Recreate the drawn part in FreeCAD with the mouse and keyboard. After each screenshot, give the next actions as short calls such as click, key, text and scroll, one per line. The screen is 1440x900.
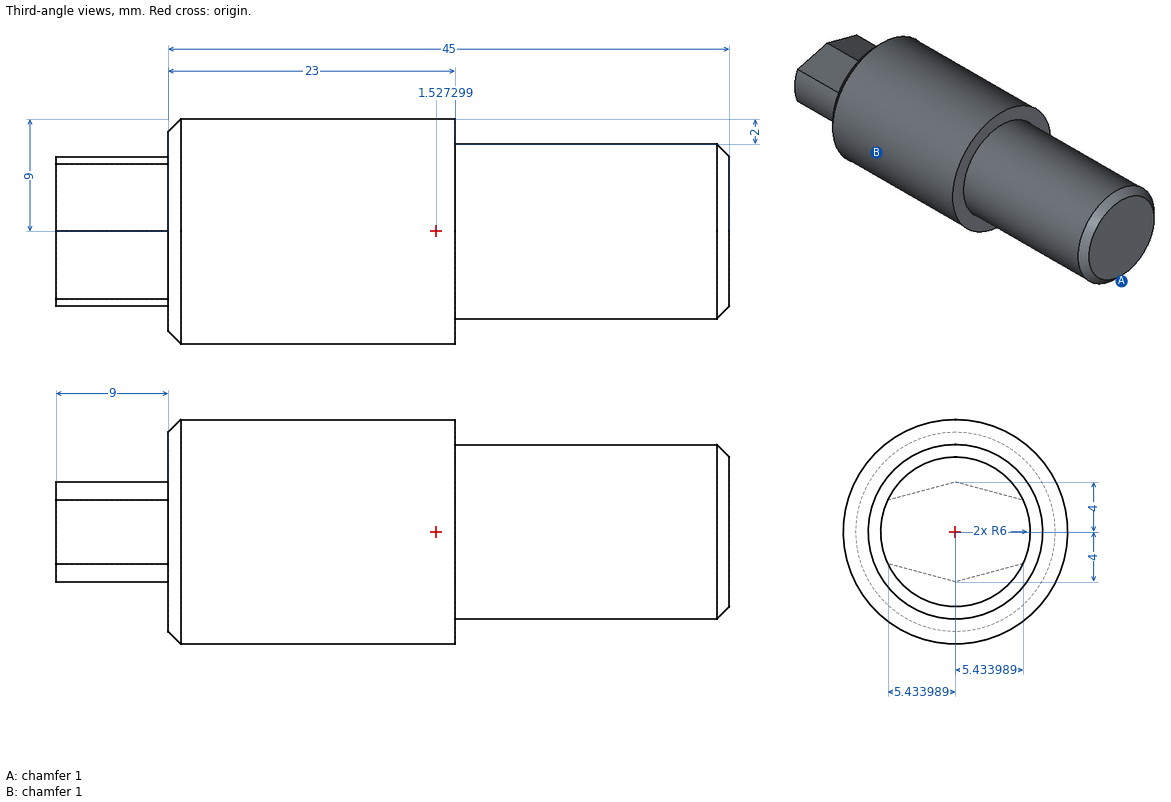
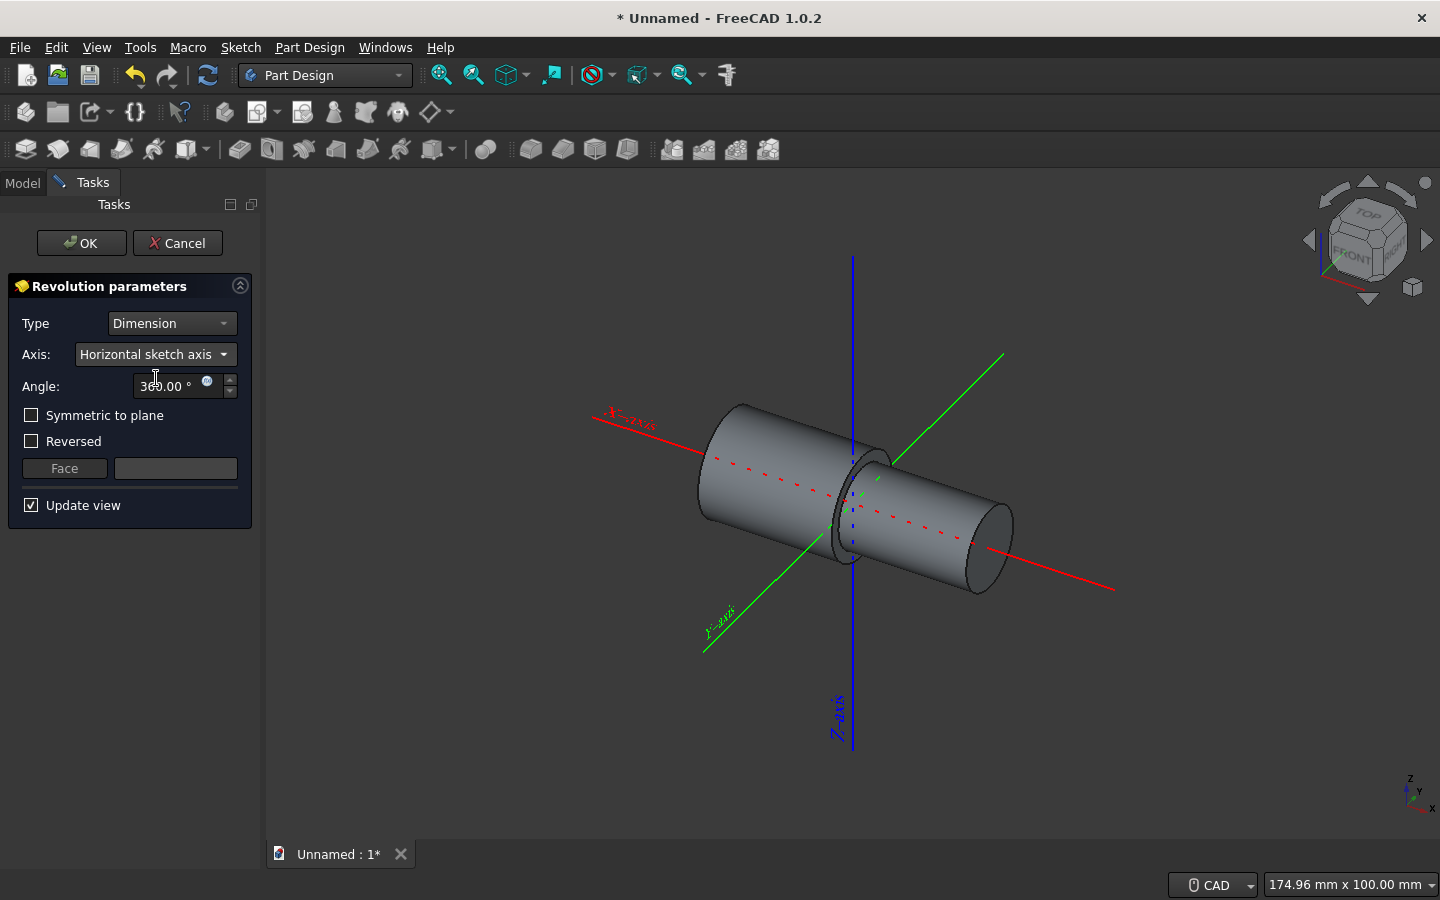
click(82, 243)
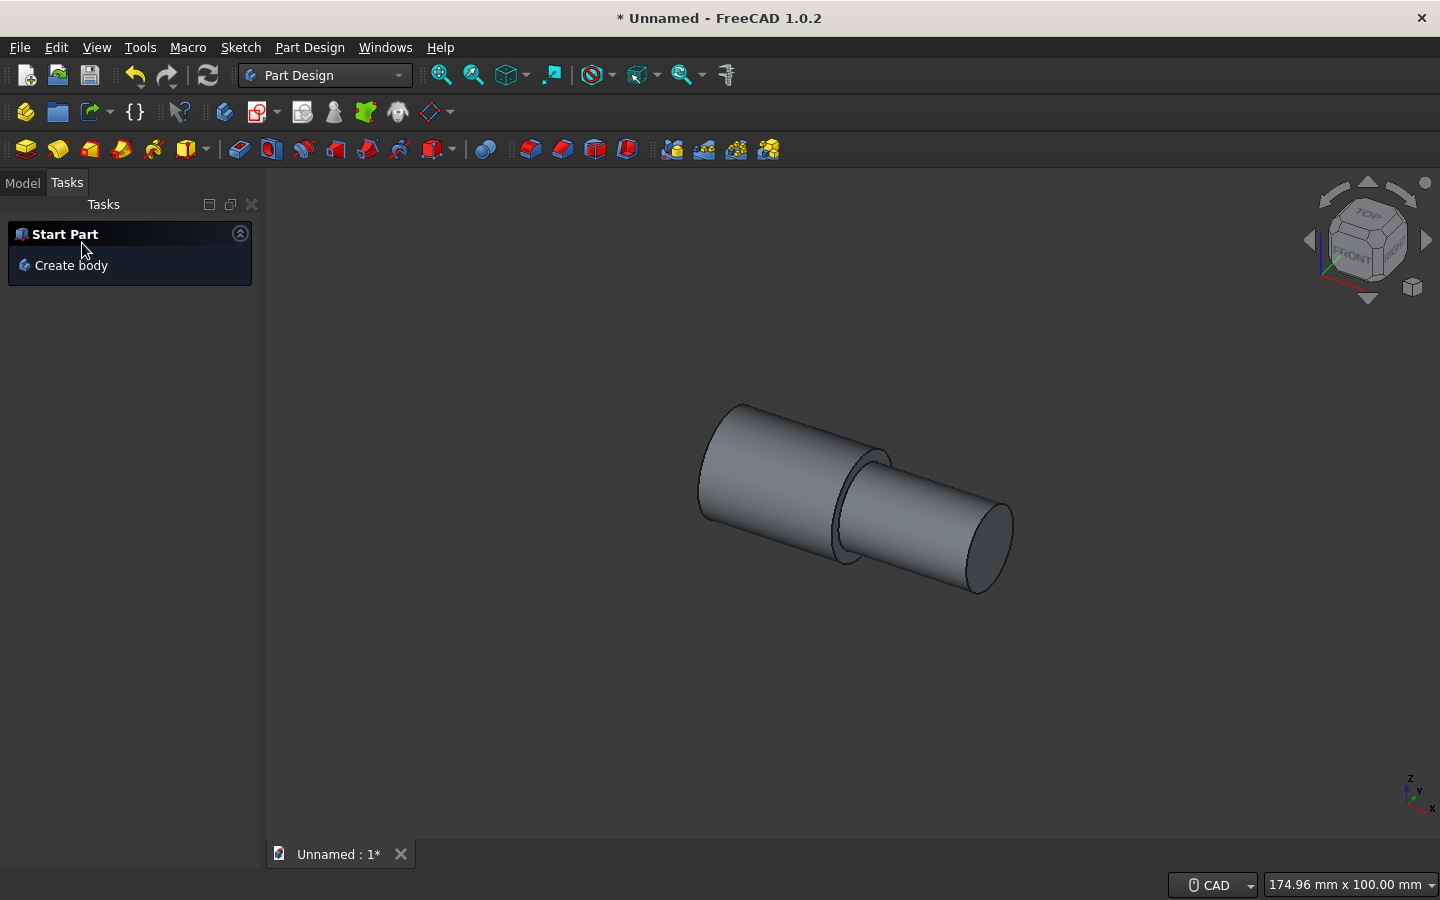
click(442, 76)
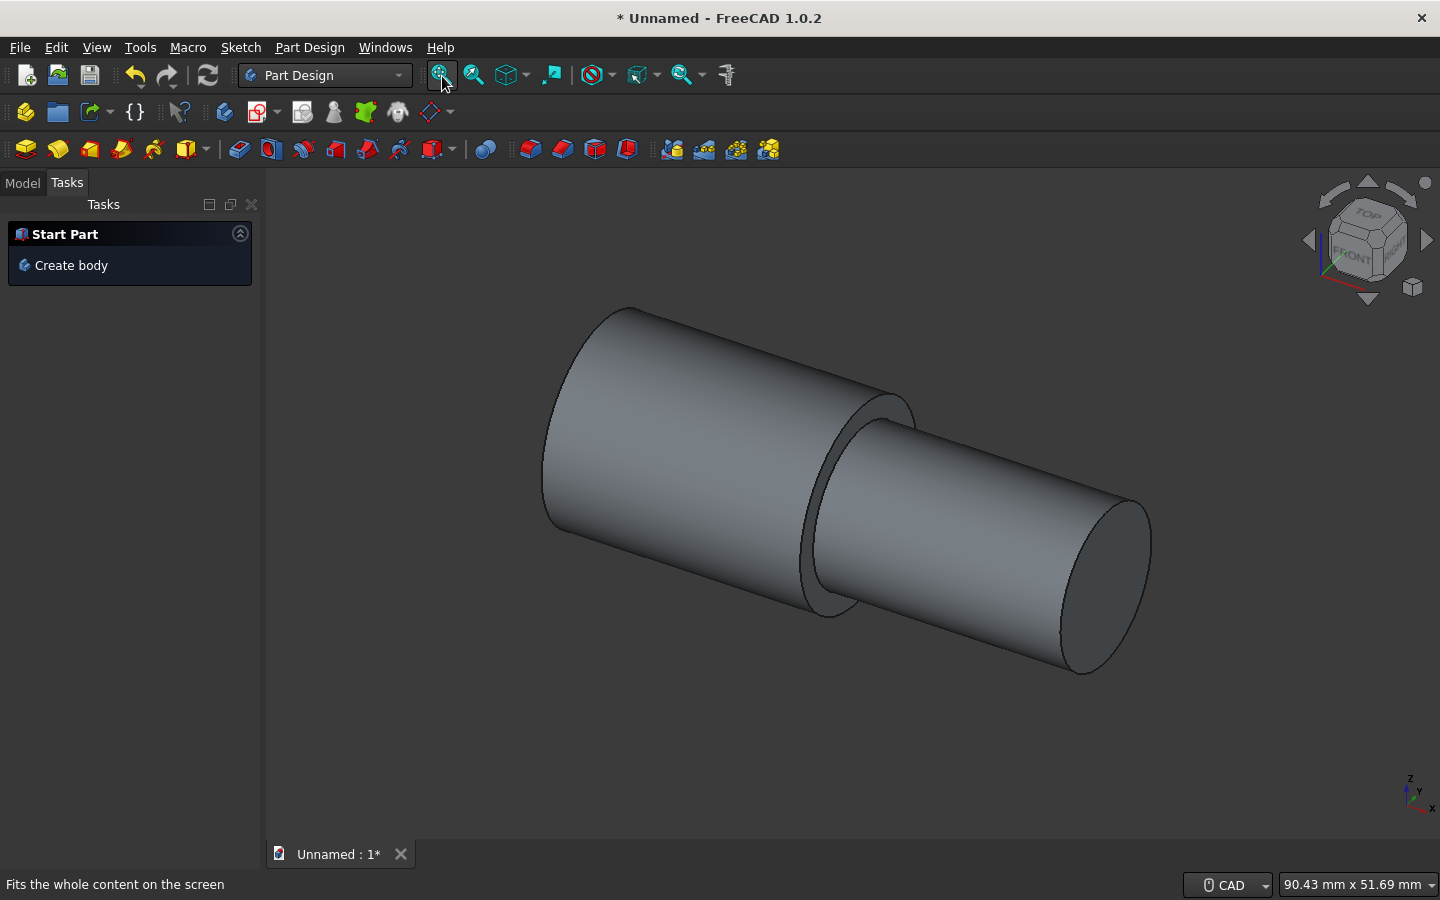
click(1060, 631)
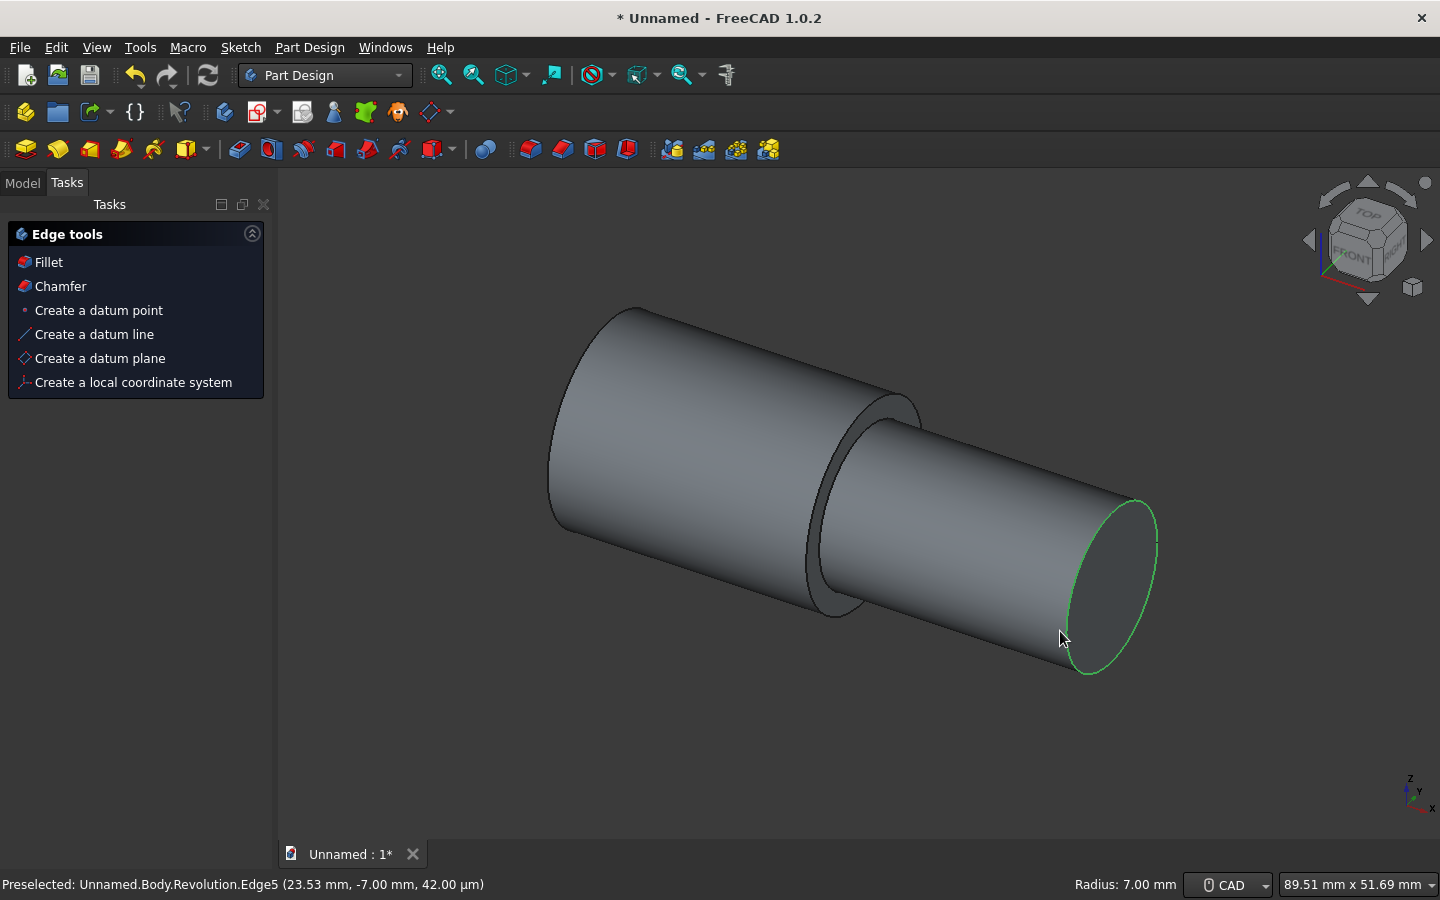
click(564, 150)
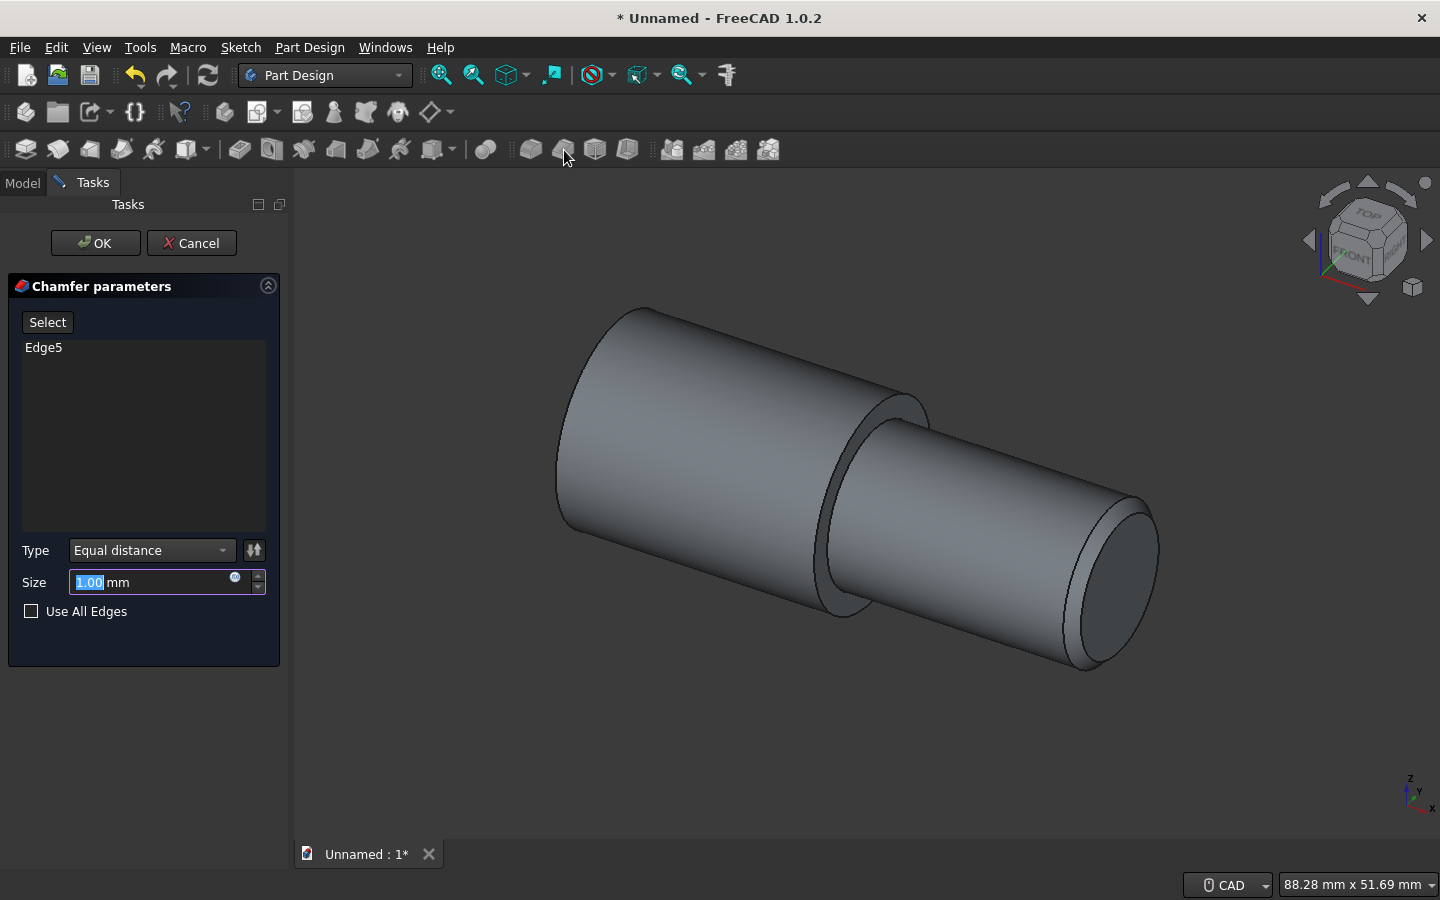
text(1)
key(Tab)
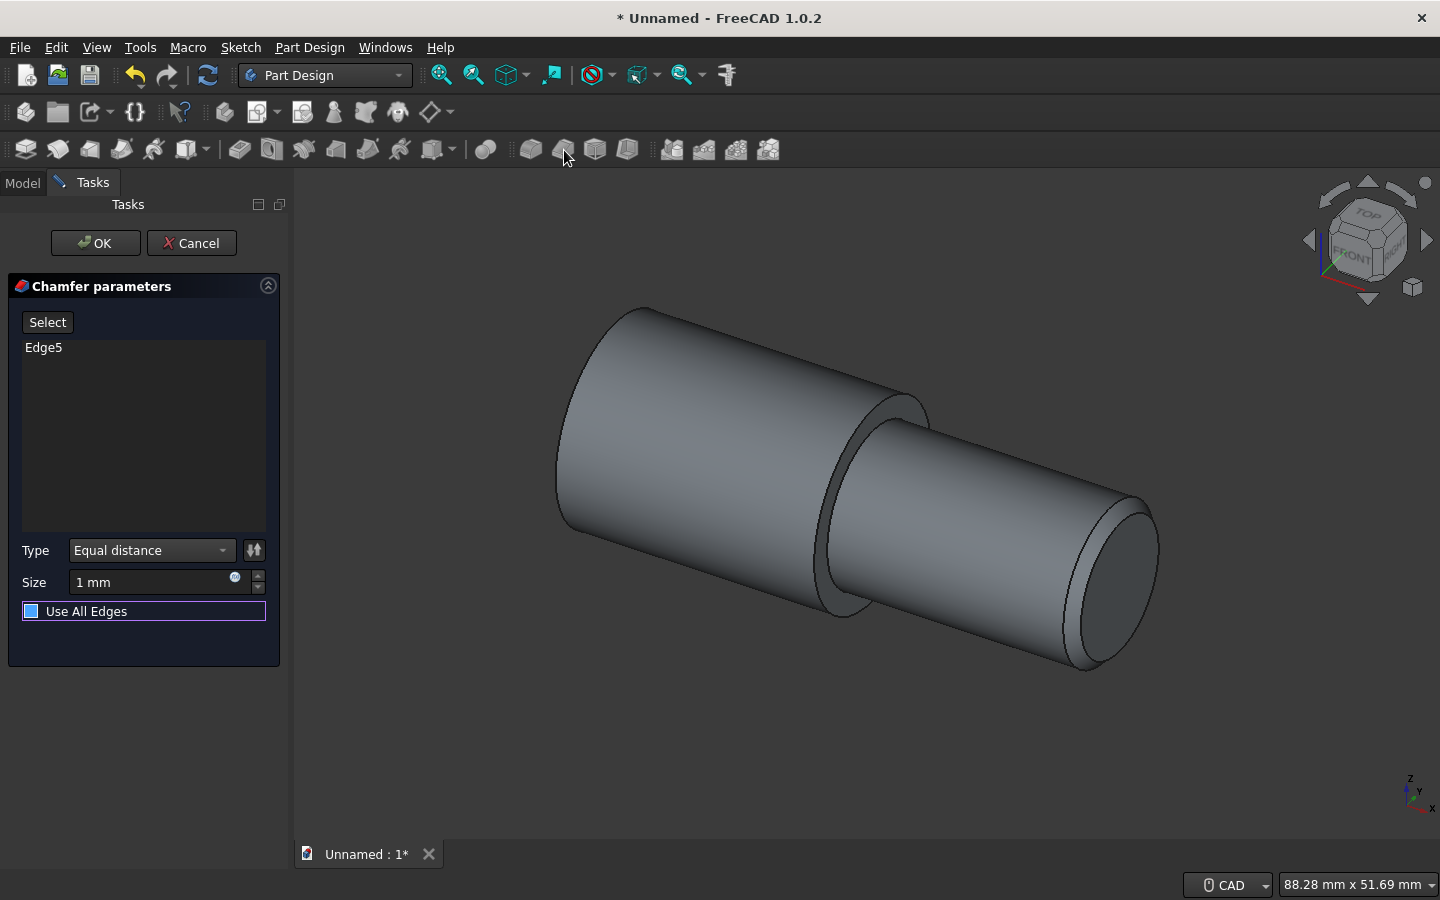
click(96, 243)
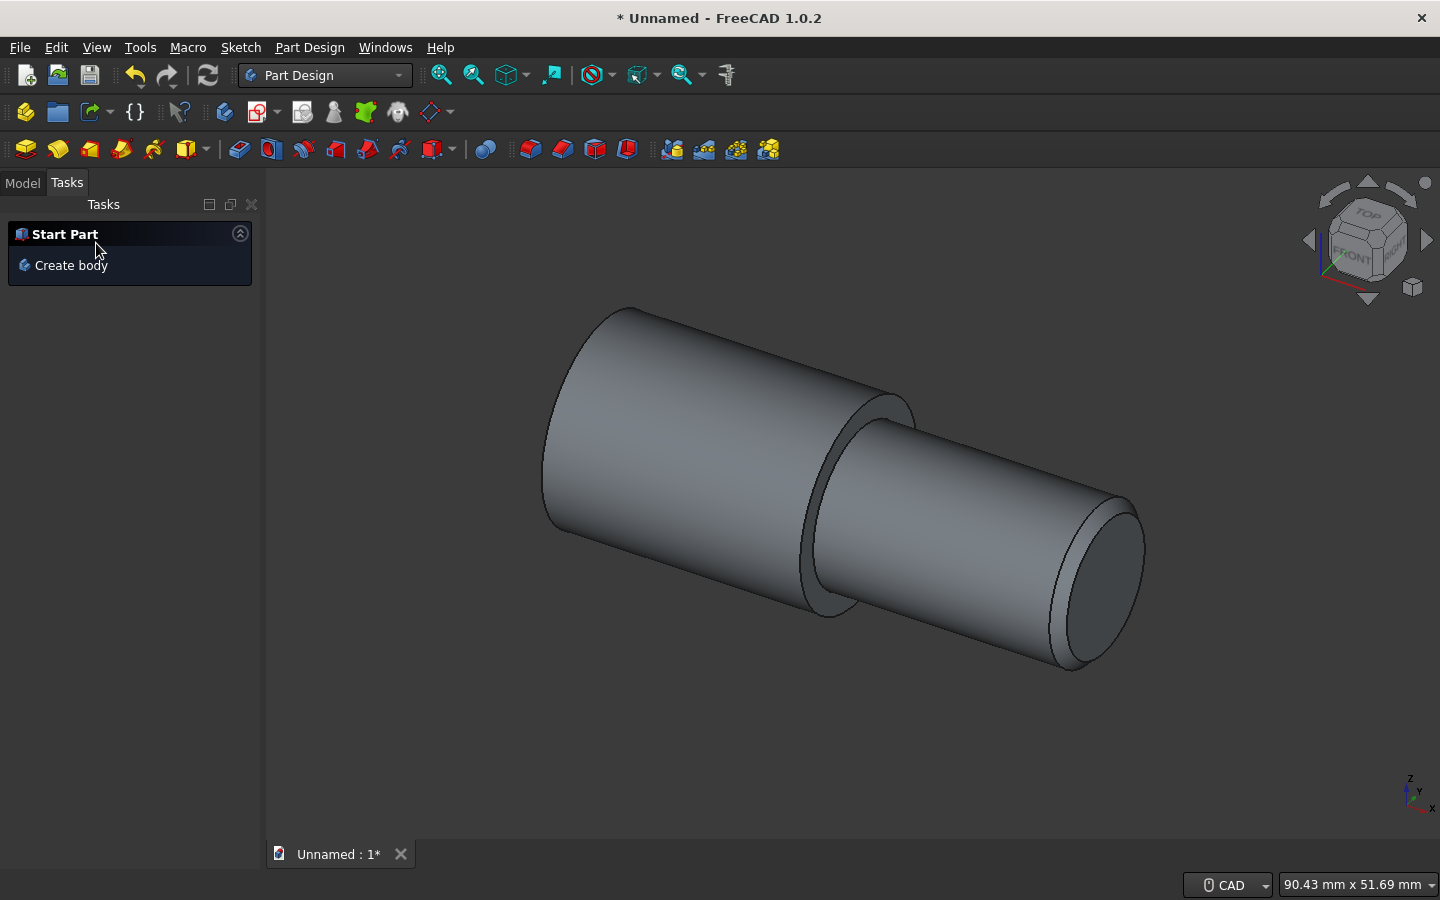
key(0)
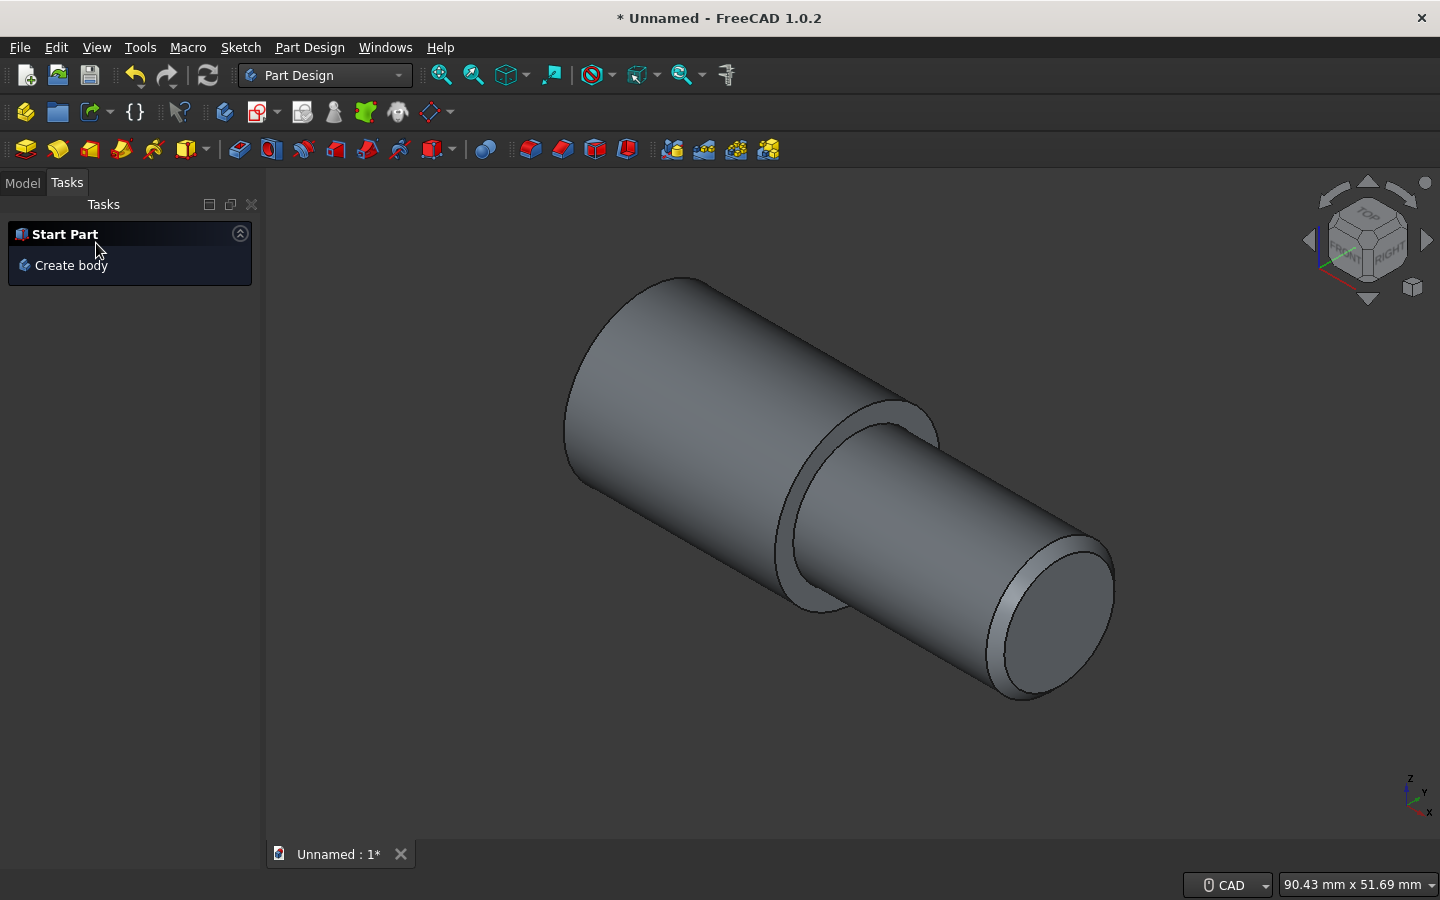
key(2)